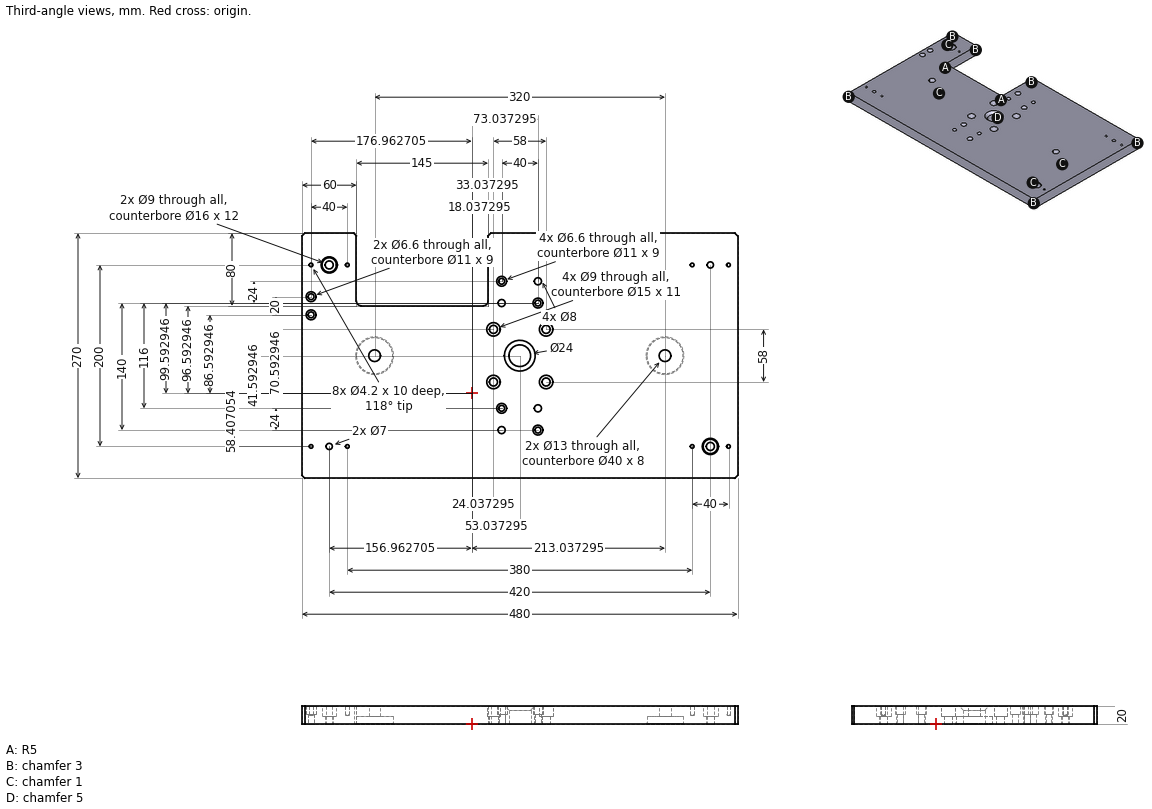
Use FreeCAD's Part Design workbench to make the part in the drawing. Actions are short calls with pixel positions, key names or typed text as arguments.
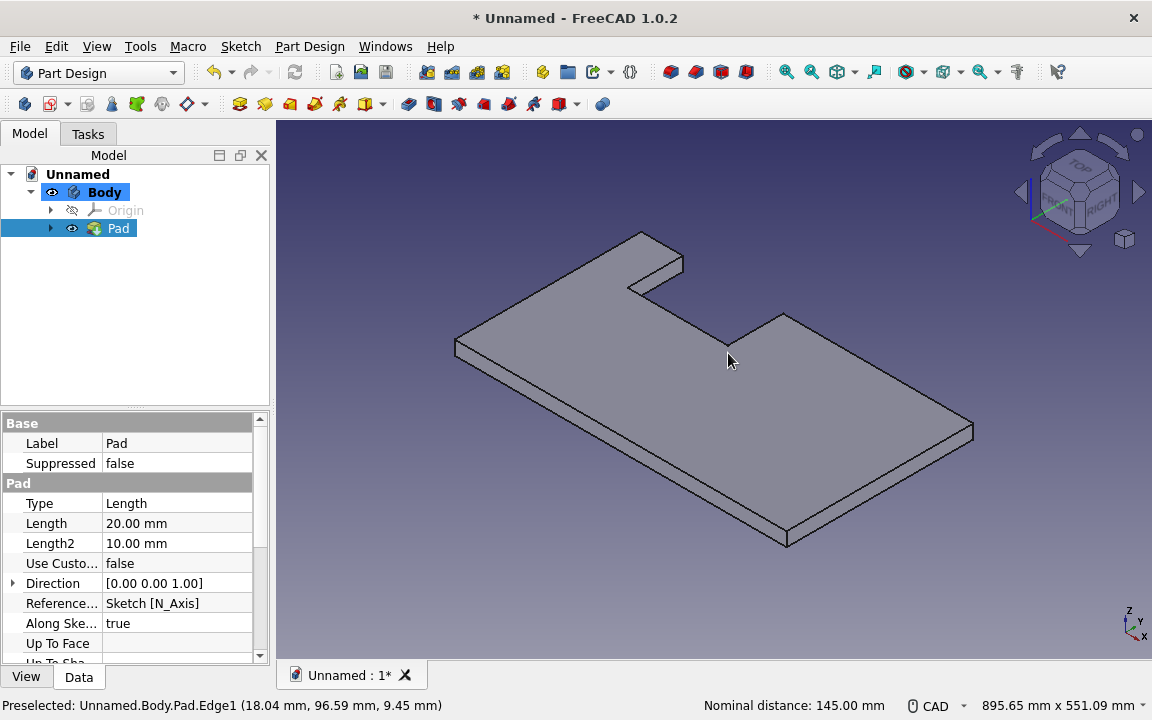
click(671, 72)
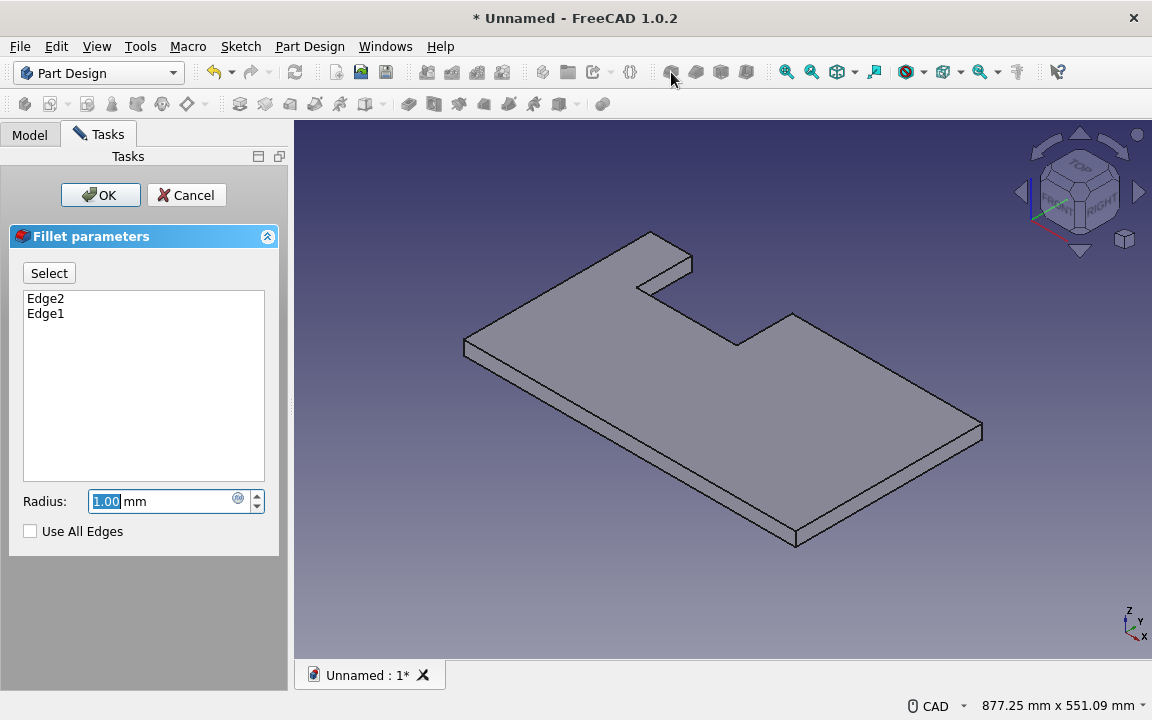
text(5)
key(Tab)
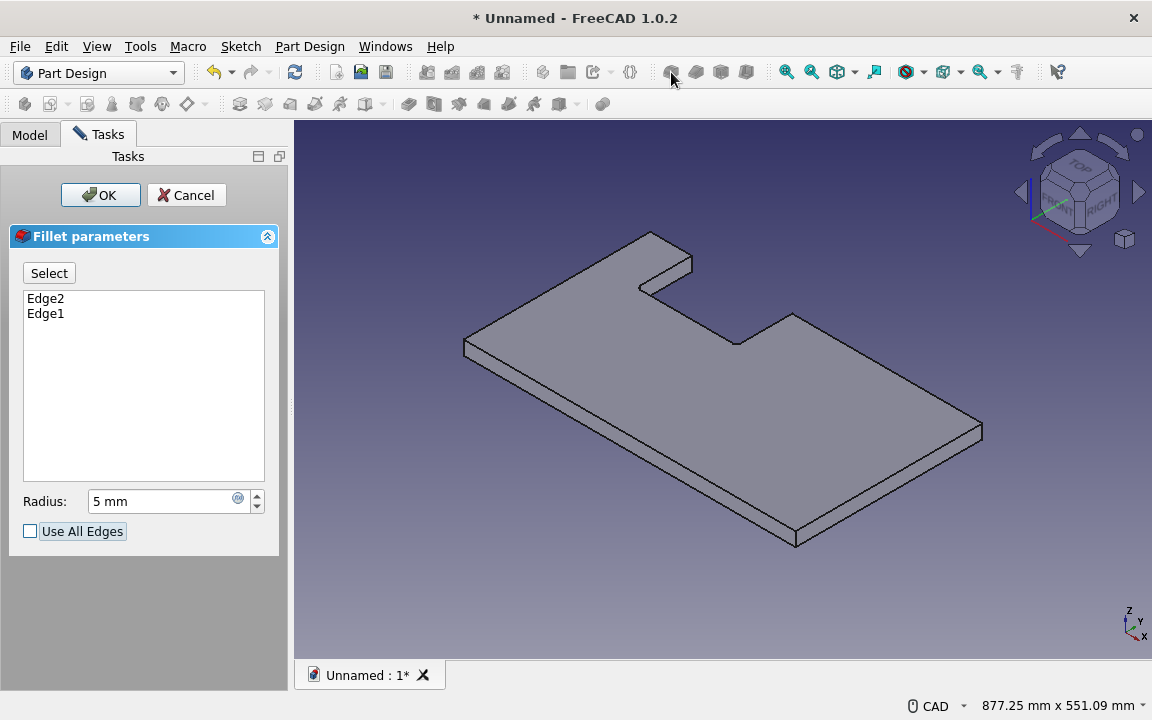
click(101, 195)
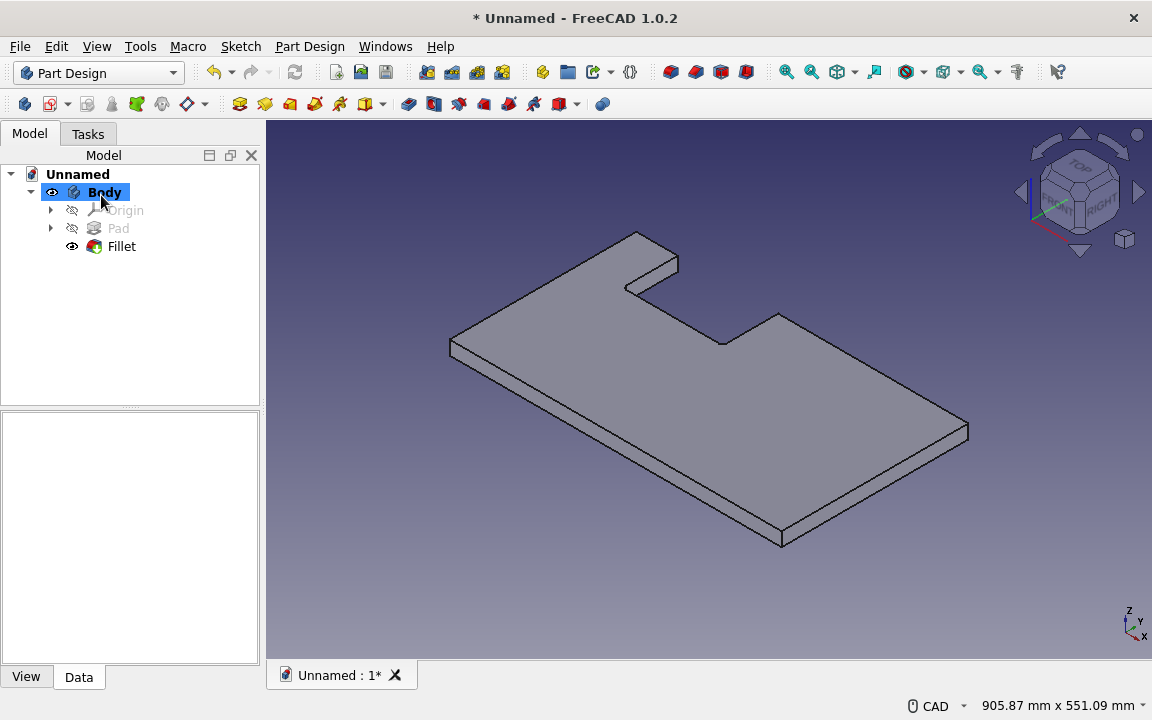
click(782, 538)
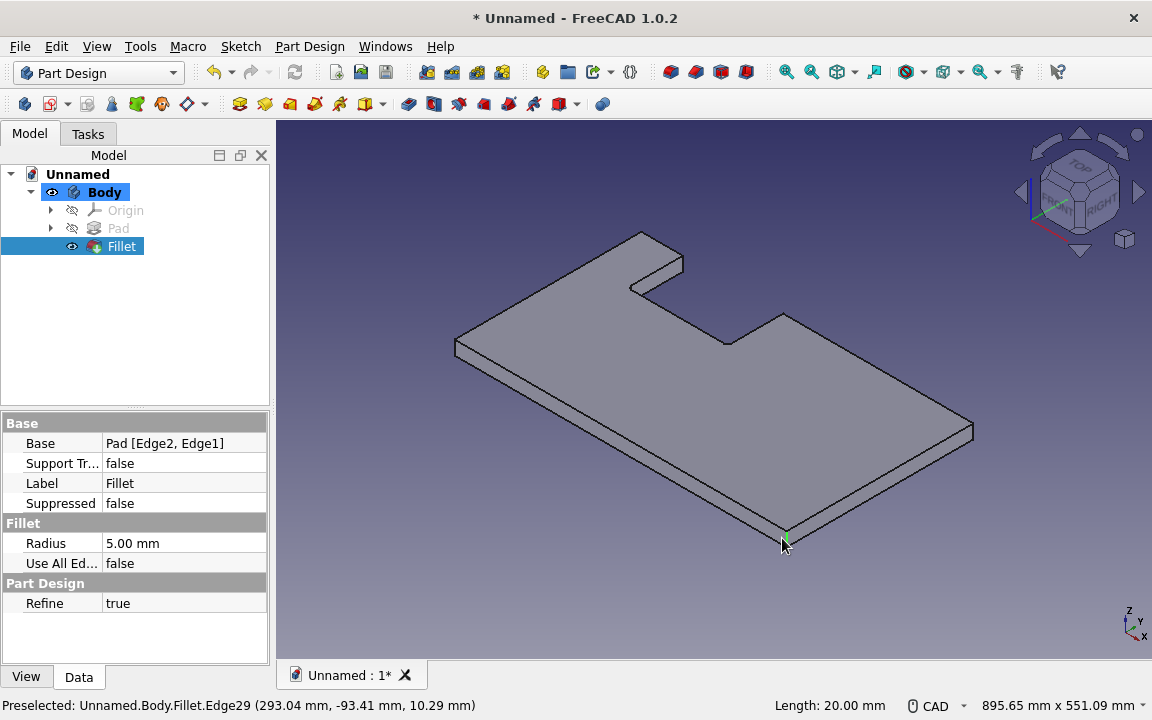
scroll(641, 239, up, 4)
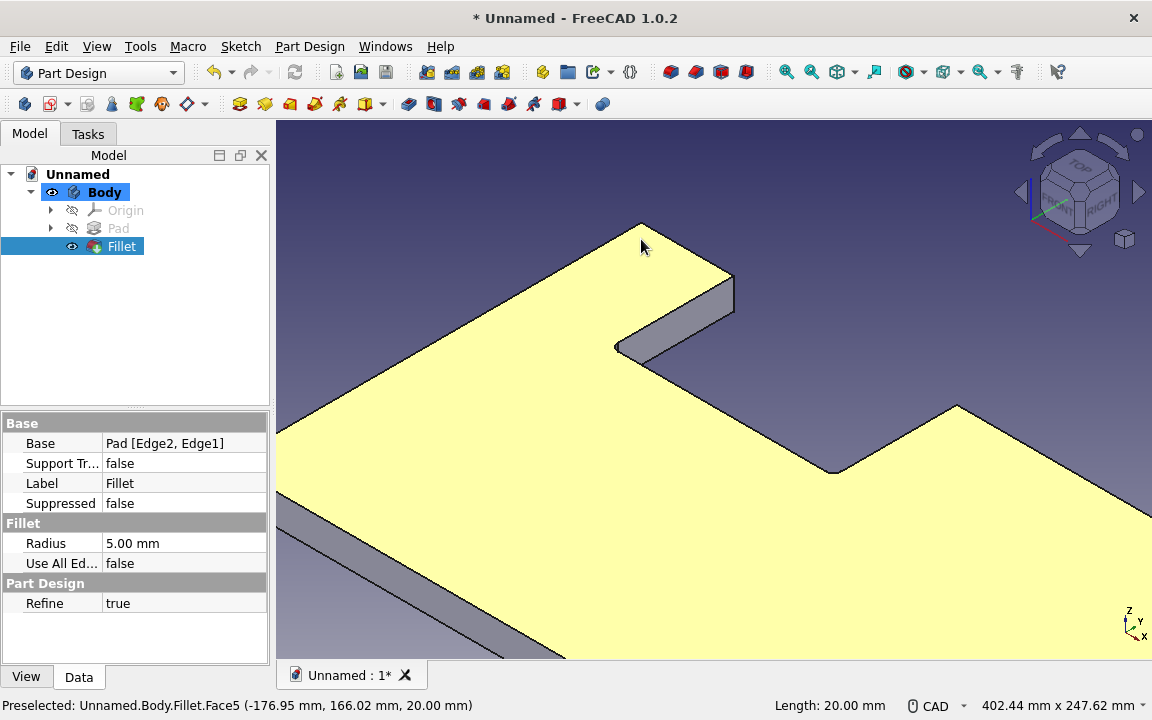
key(v)
key(f)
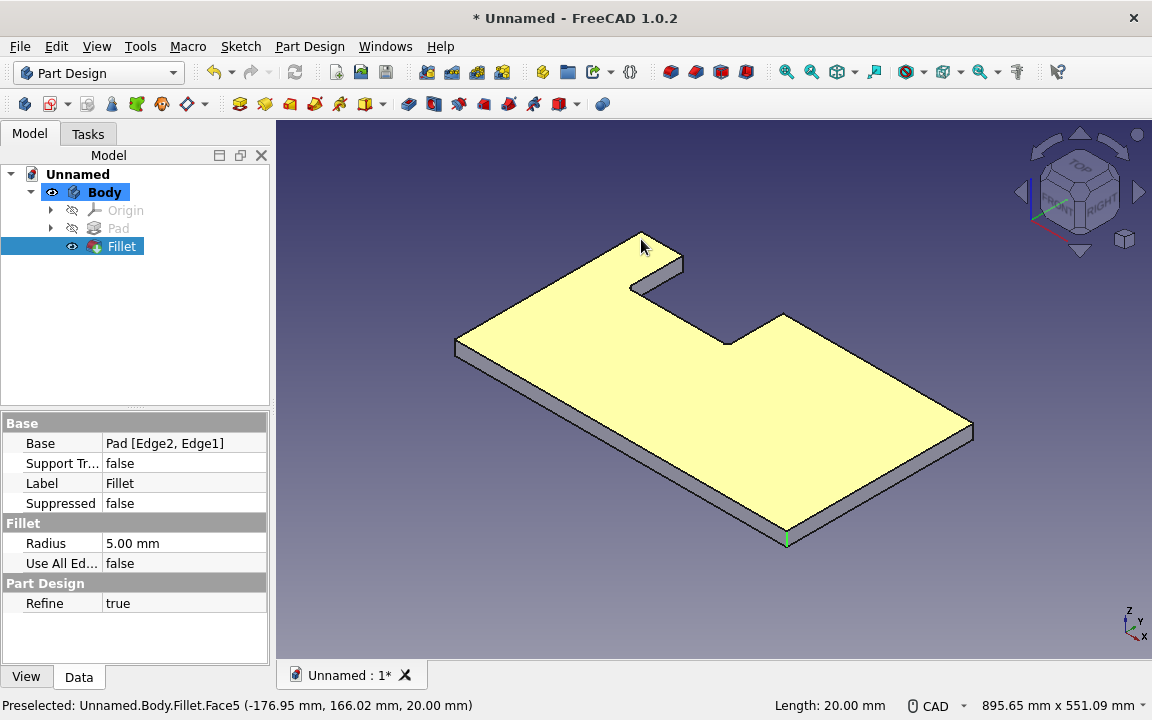
key(2)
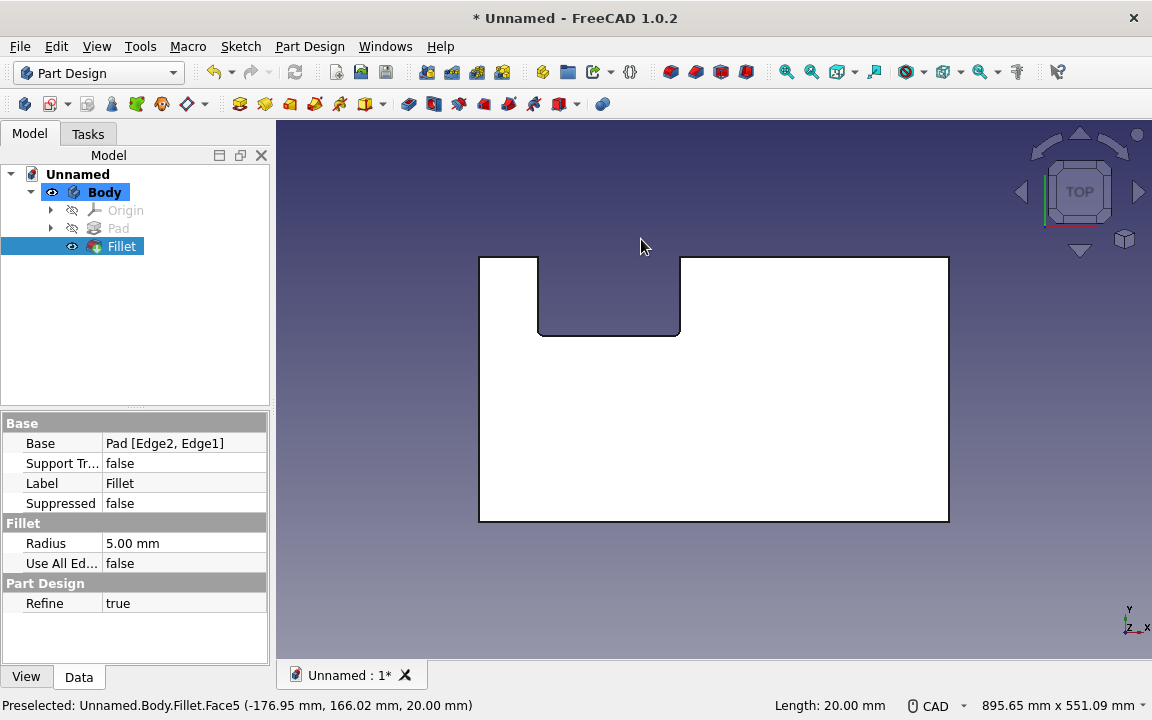
scroll(479, 256, up, 4)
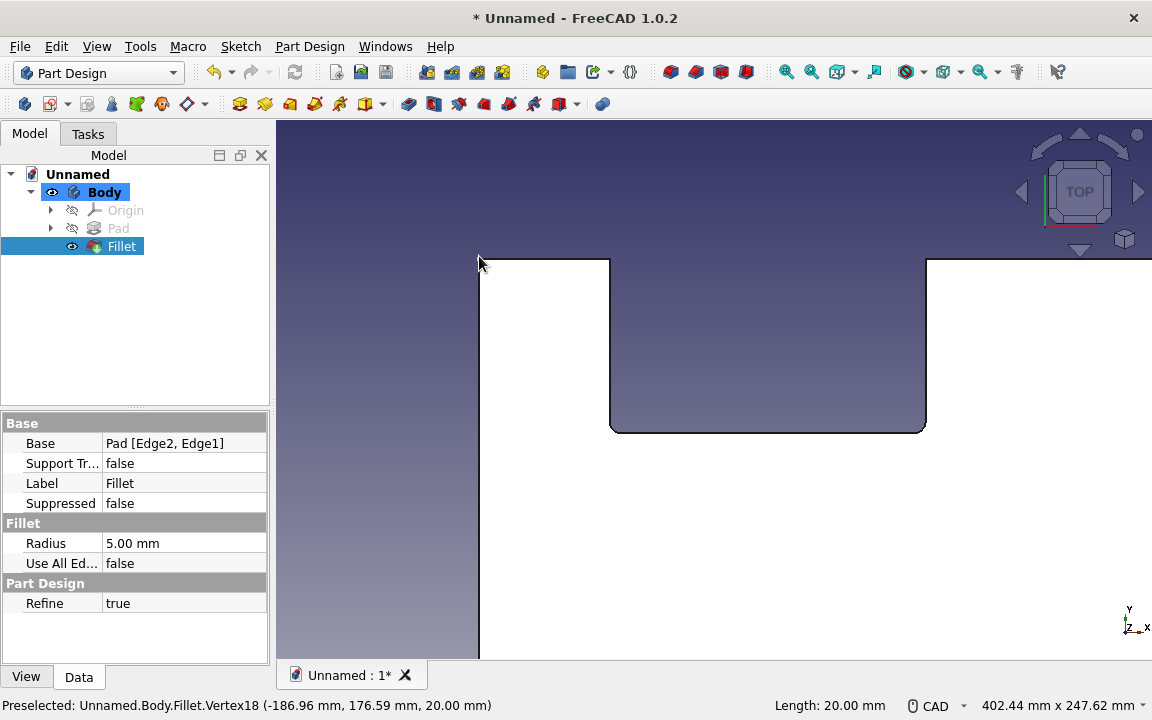
click(787, 72)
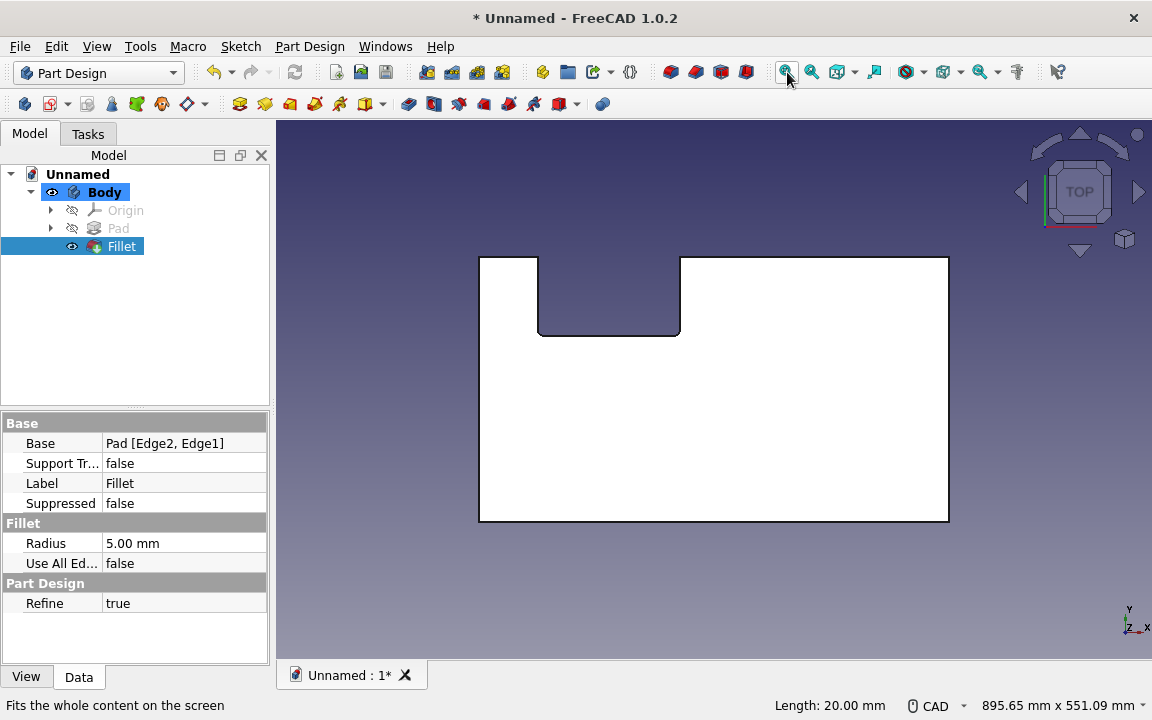
key(0)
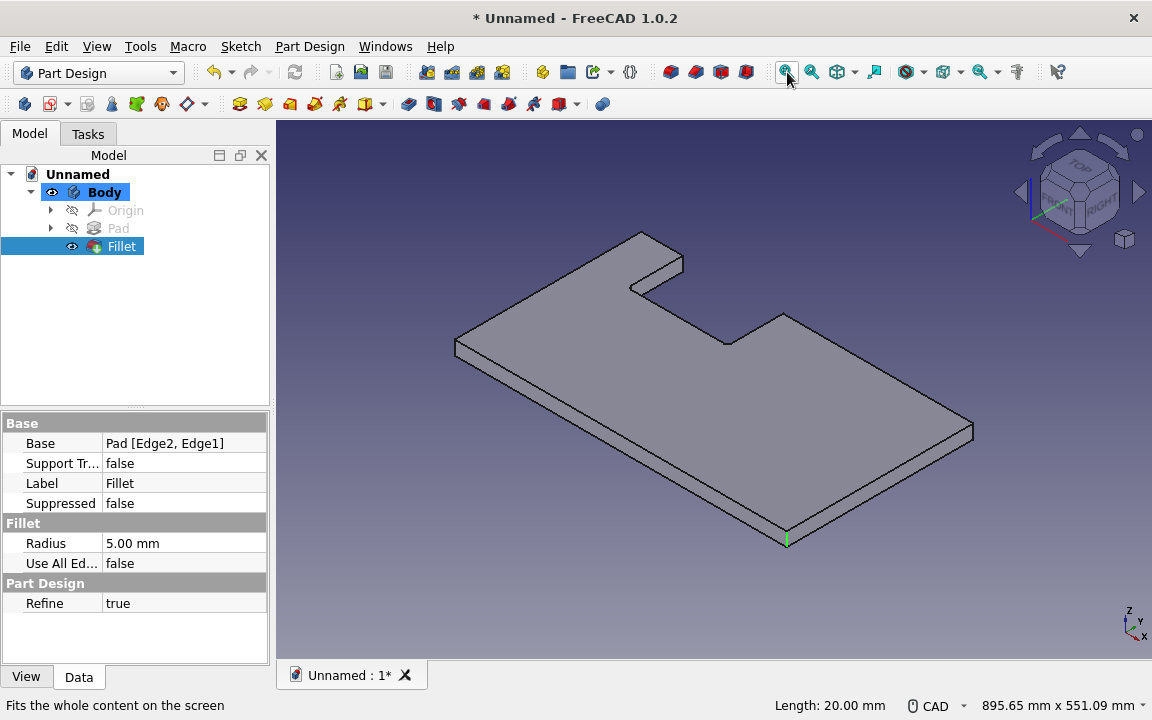
scroll(641, 239, up, 4)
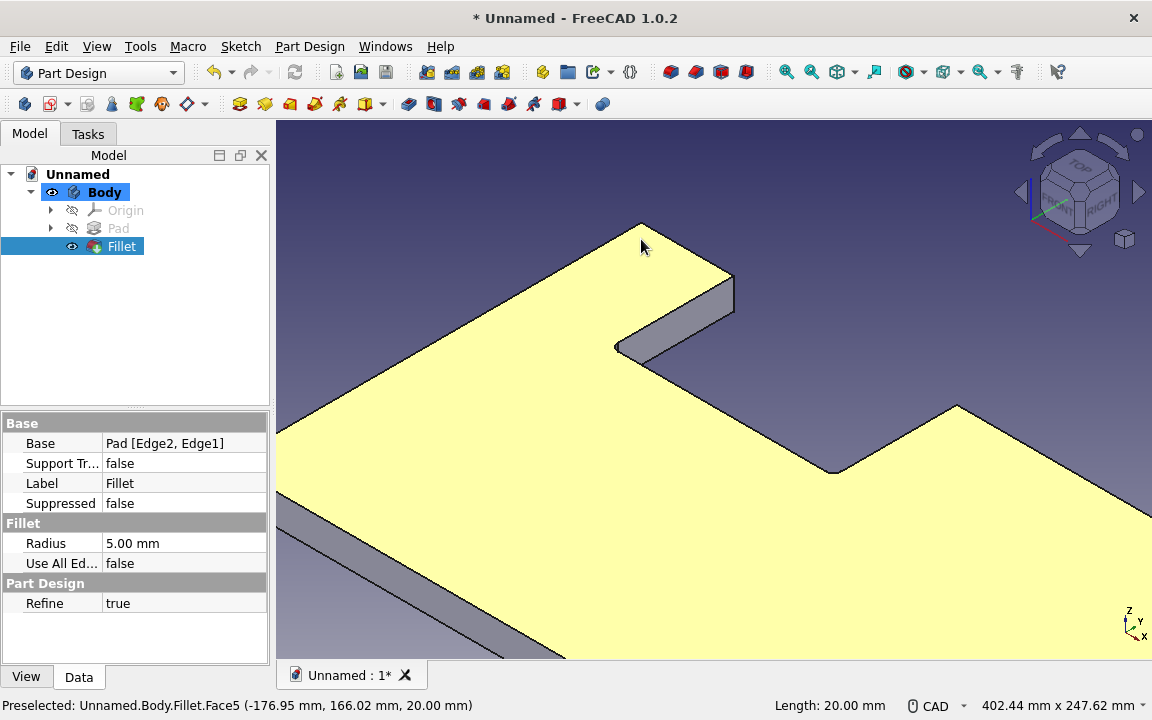
key(v)
key(f)